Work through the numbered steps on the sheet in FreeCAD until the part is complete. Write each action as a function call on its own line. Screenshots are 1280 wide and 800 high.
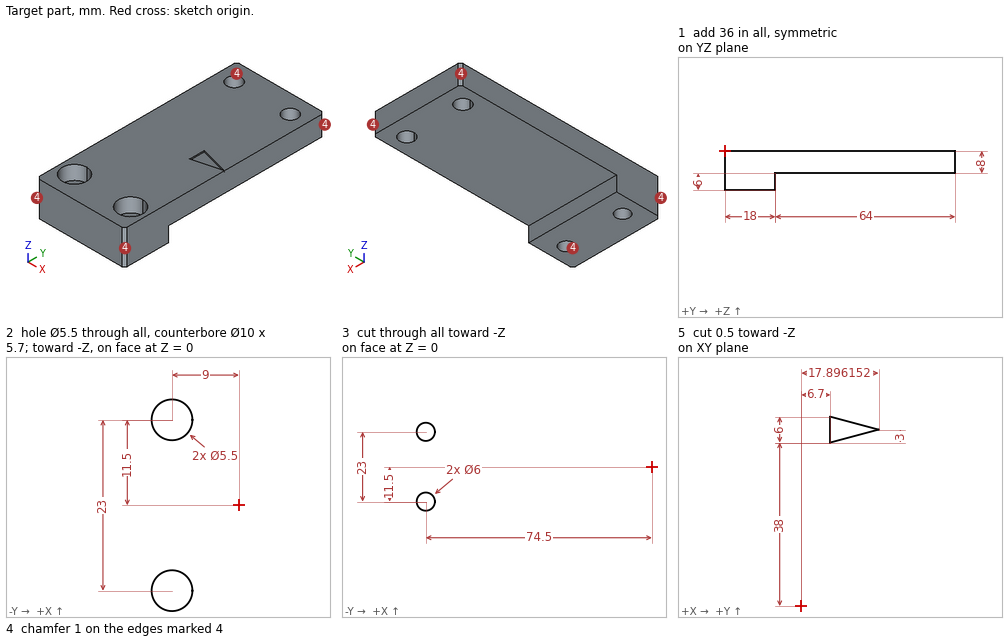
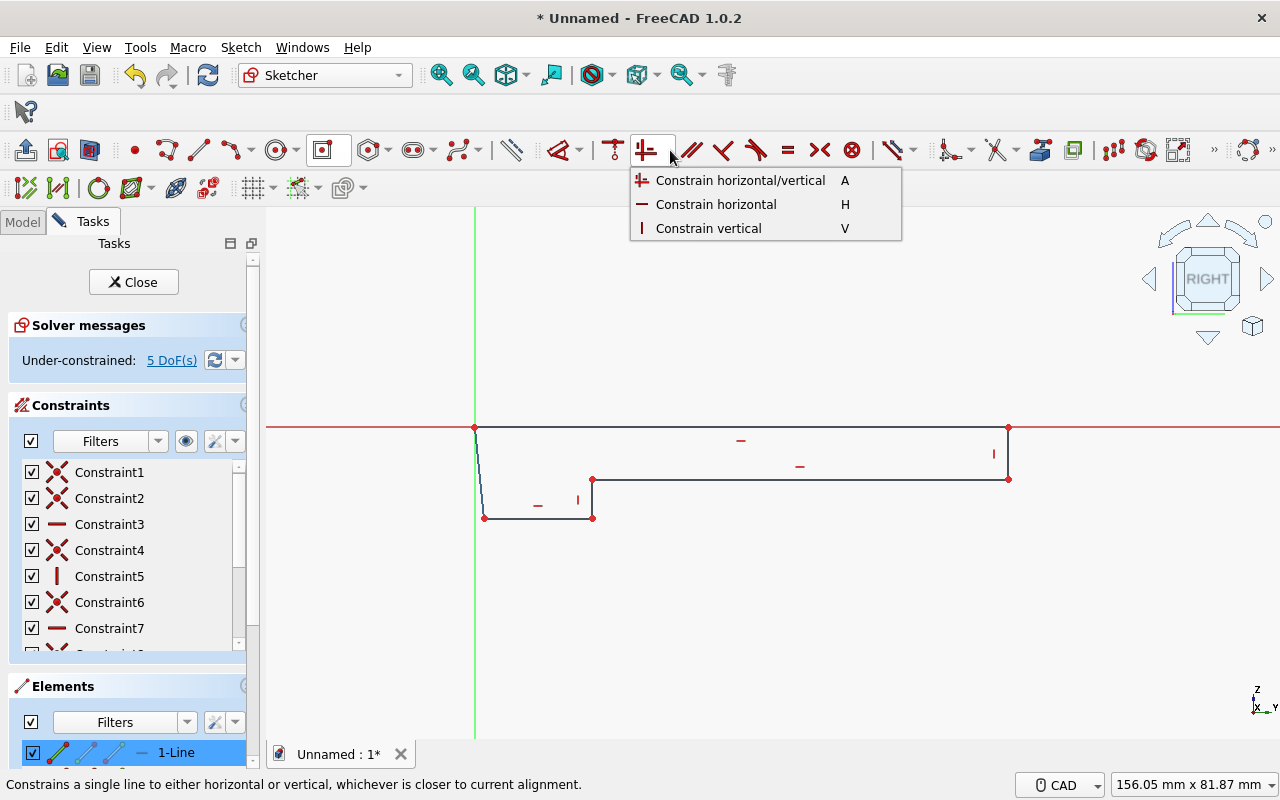
click(766, 228)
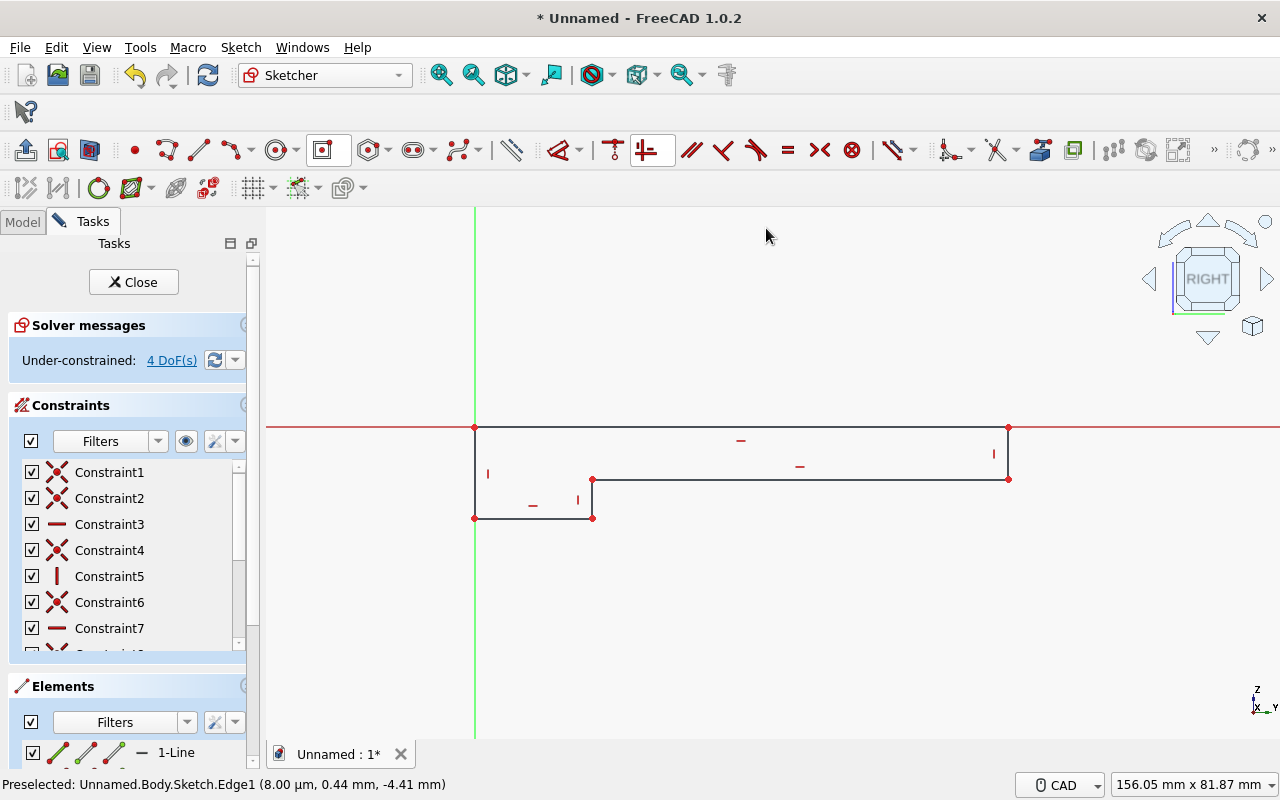
click(558, 150)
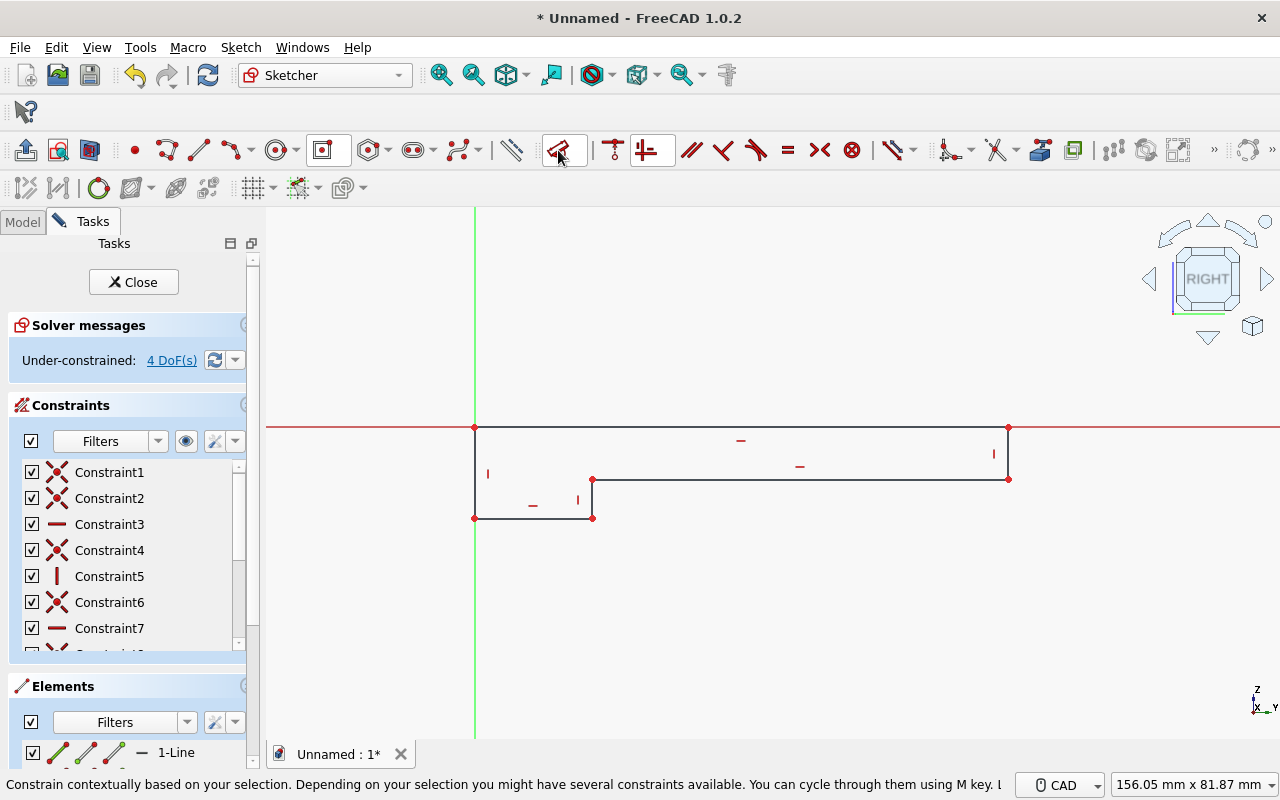
click(592, 507)
click(558, 500)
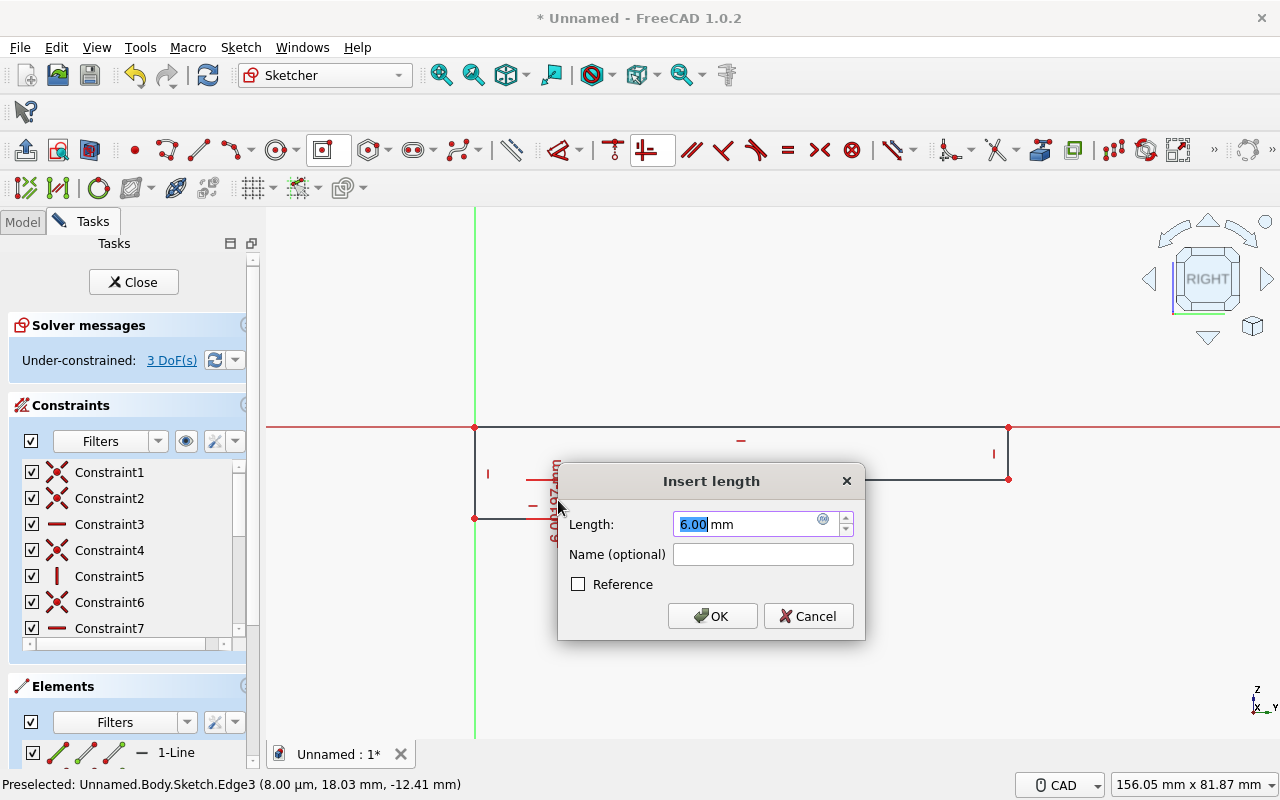
text(6)
key(Return)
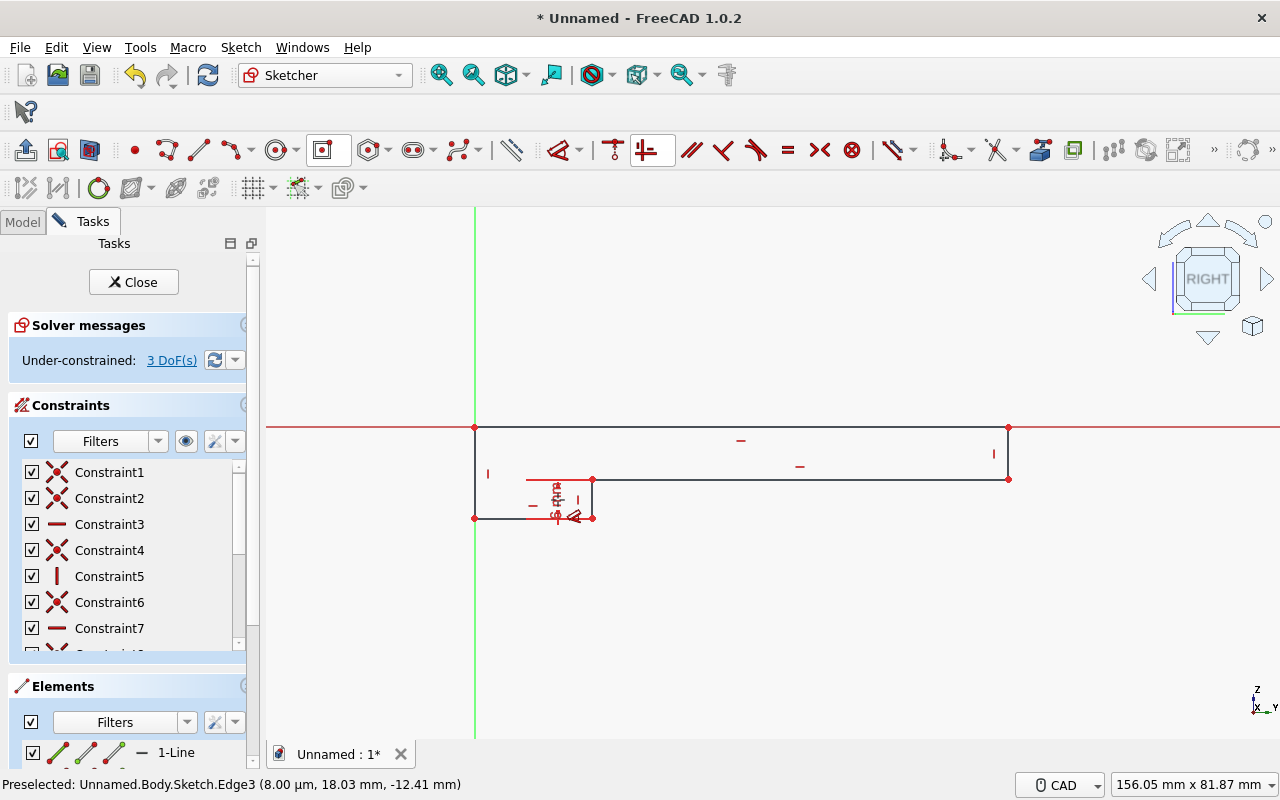
click(1008, 464)
click(1042, 454)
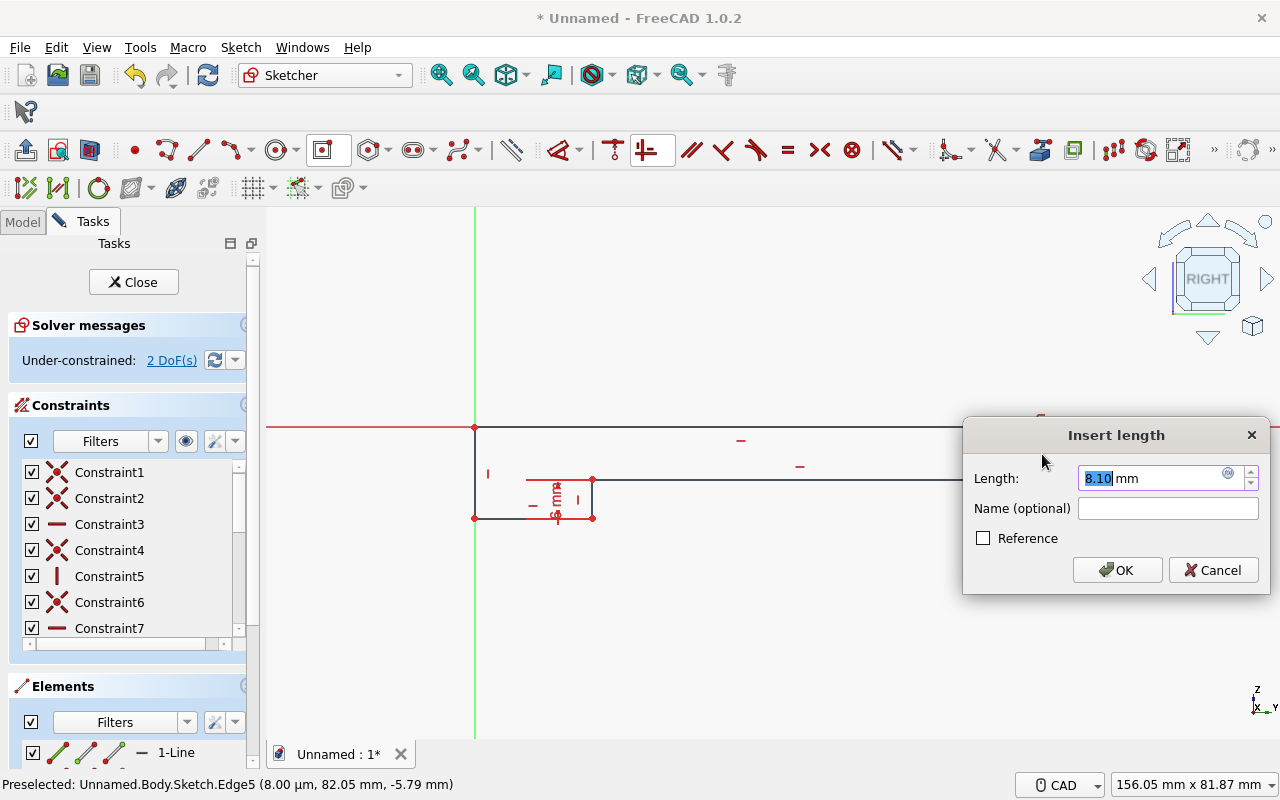
text(8)
key(Return)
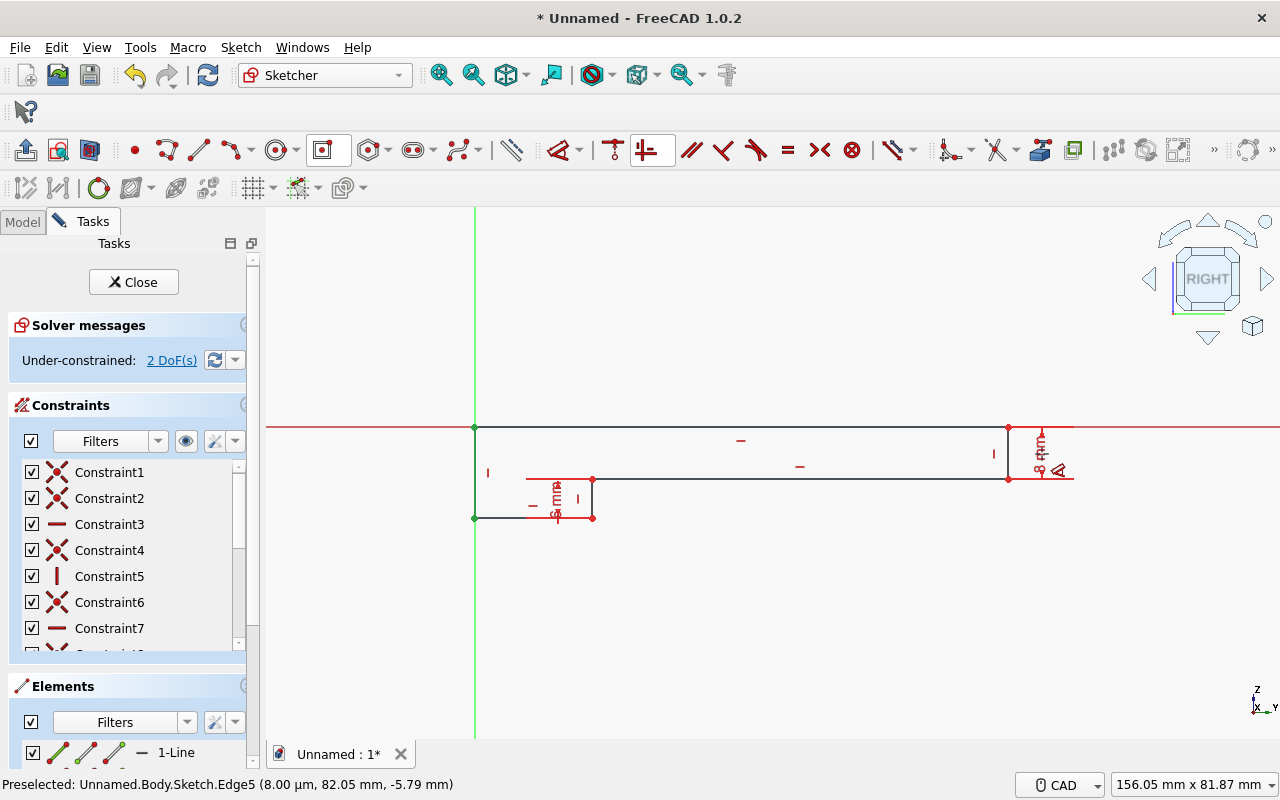
click(510, 518)
click(533, 552)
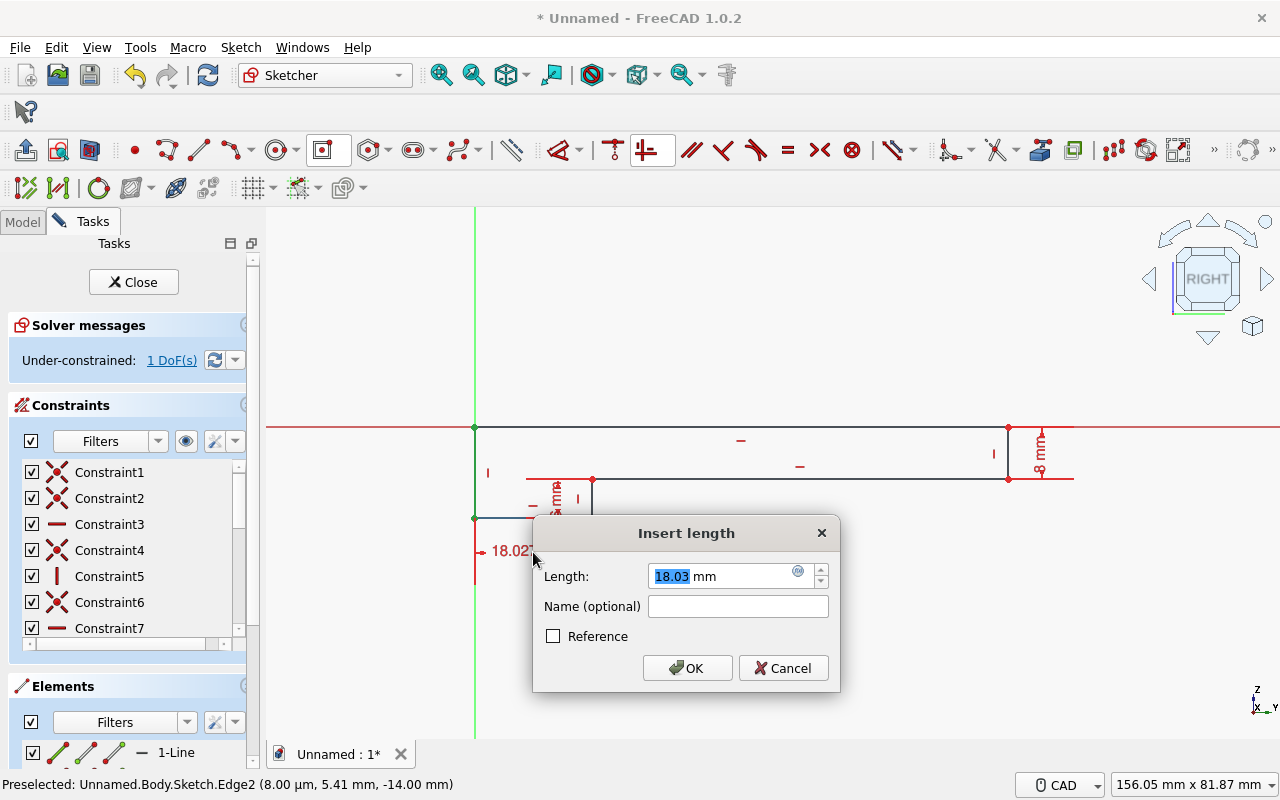
text(18)
key(Return)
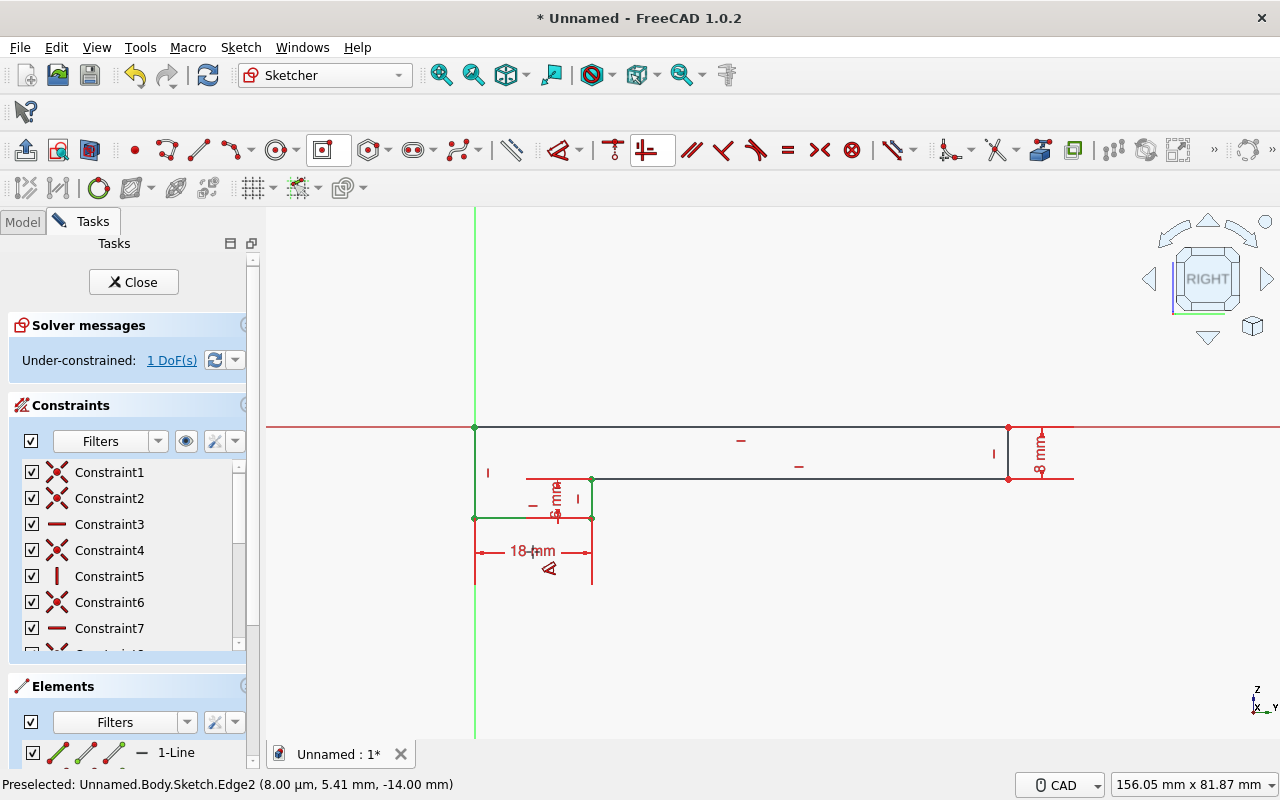
click(717, 479)
click(800, 513)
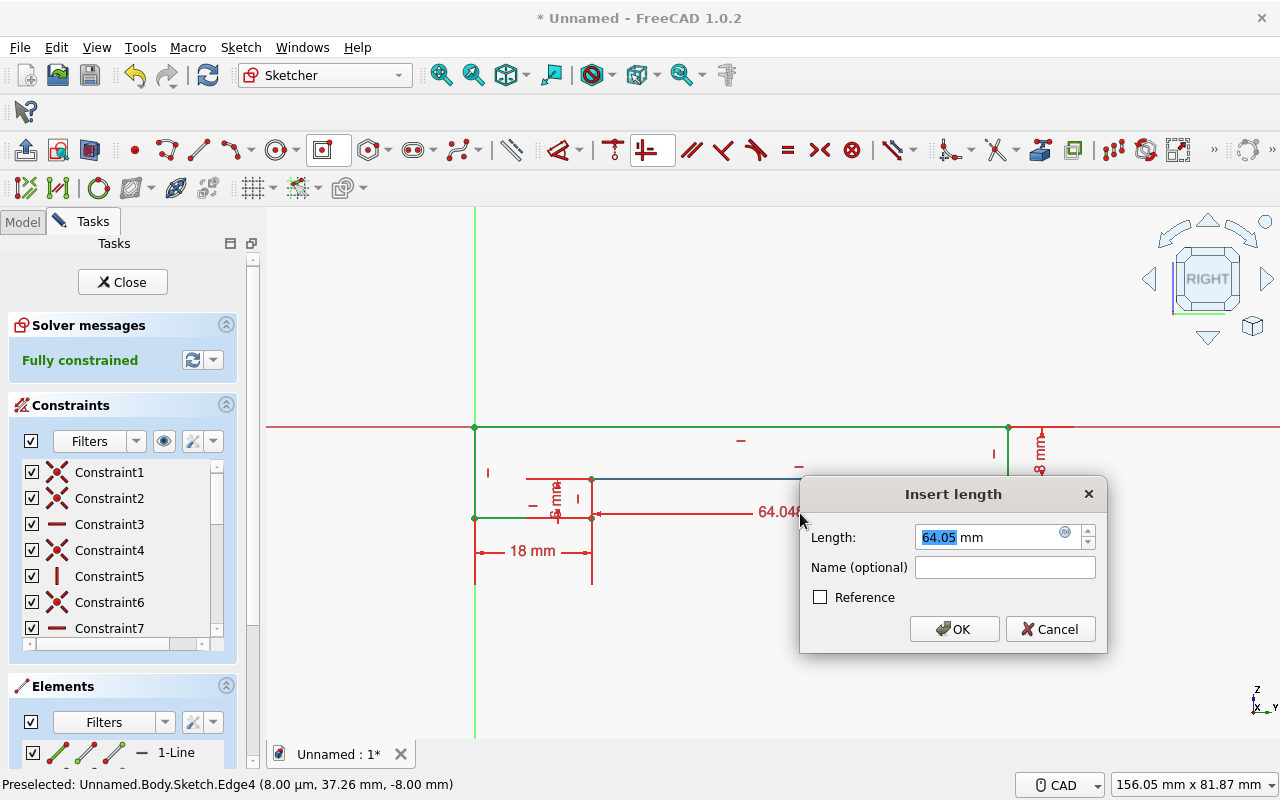
text(64)
key(Return)
key(Escape)